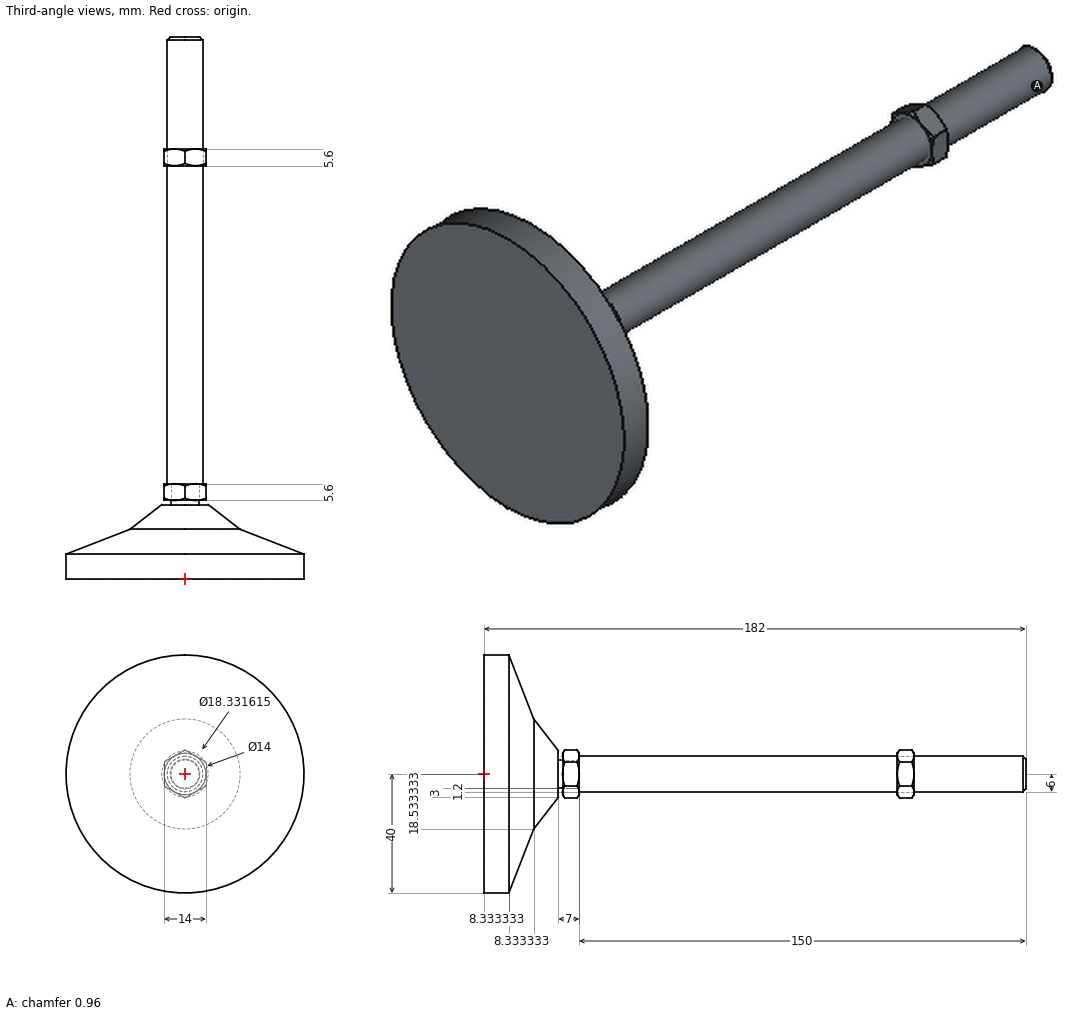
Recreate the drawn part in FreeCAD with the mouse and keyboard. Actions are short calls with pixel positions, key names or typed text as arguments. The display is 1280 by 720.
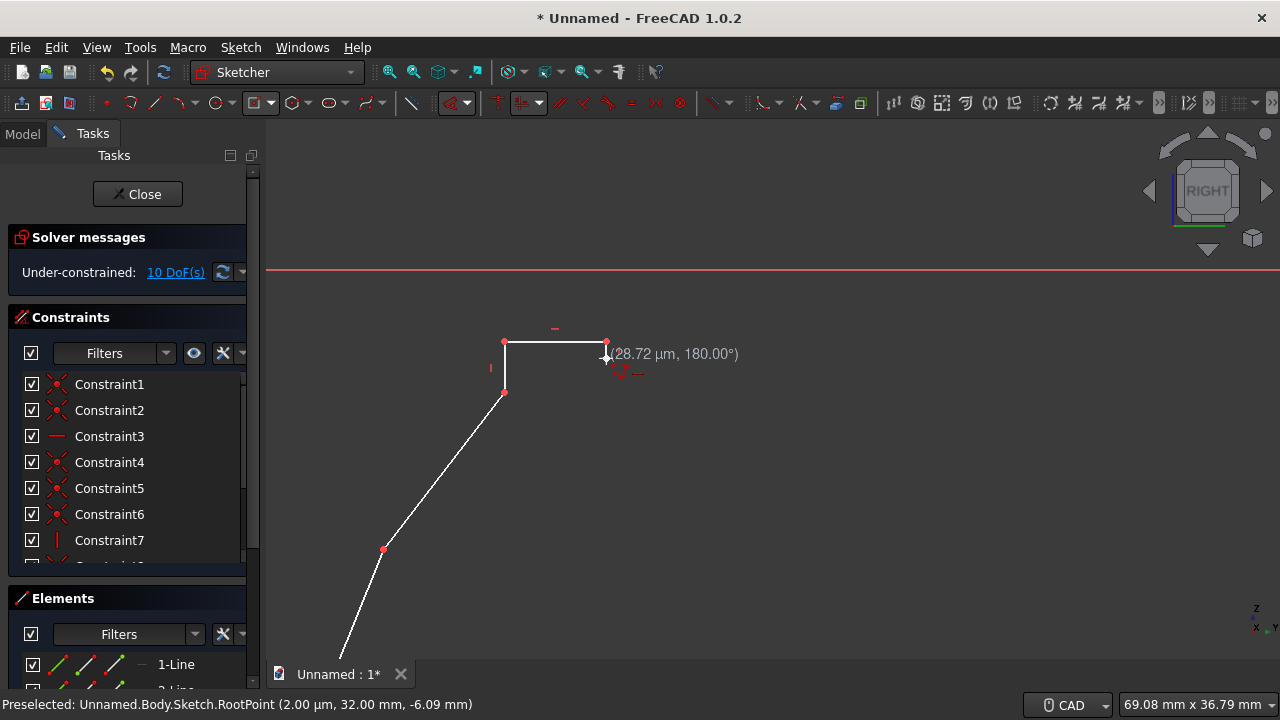
scroll(510, 345, down, 8)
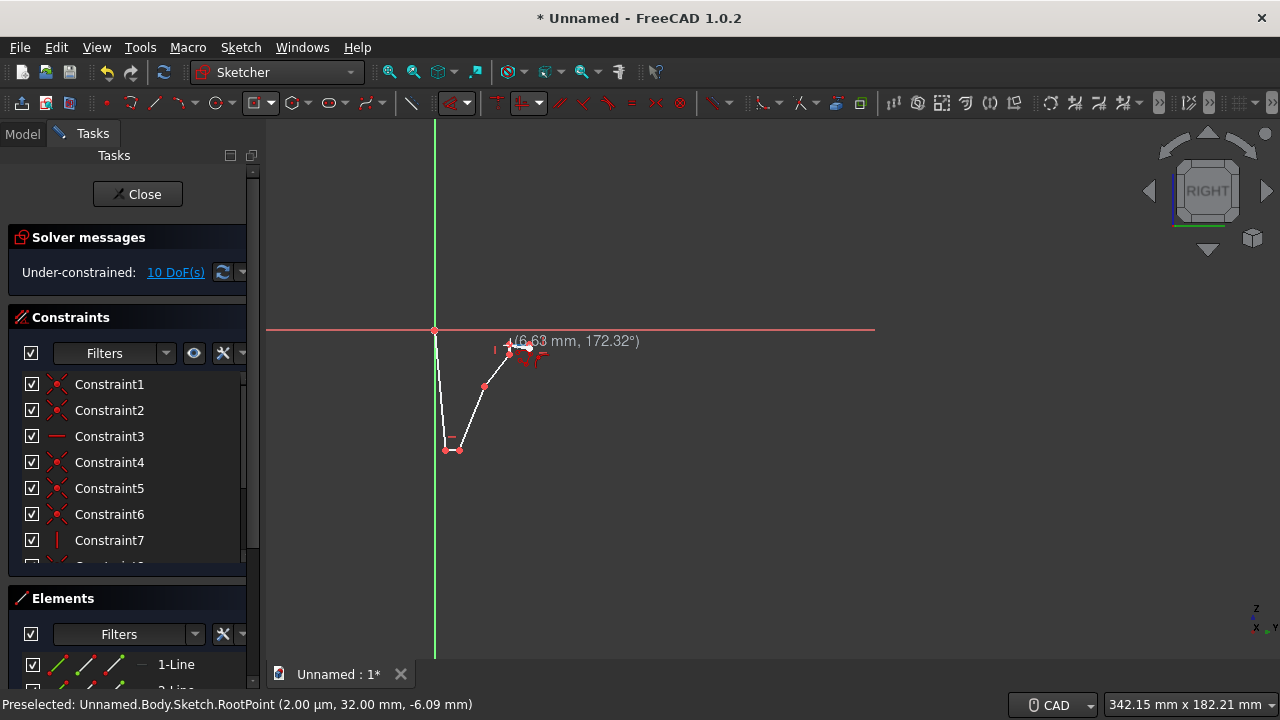
click(974, 348)
click(974, 339)
click(435, 330)
key(Escape)
key(Escape)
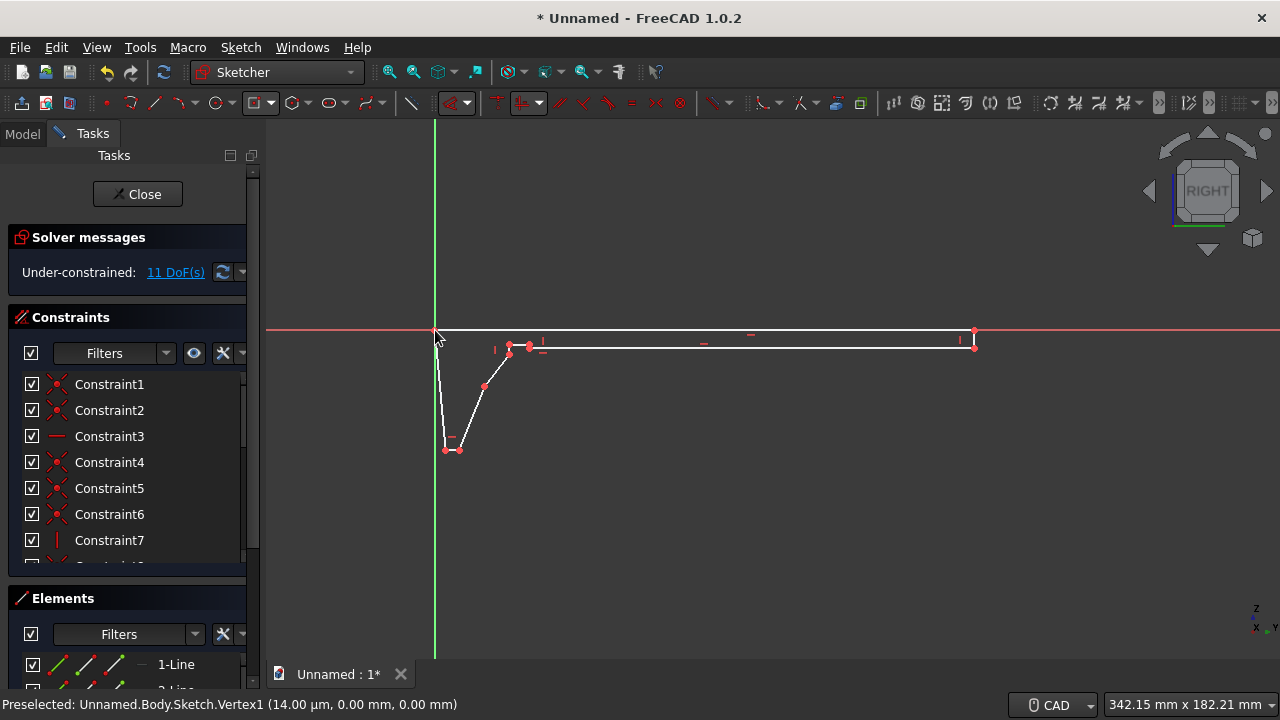
click(438, 366)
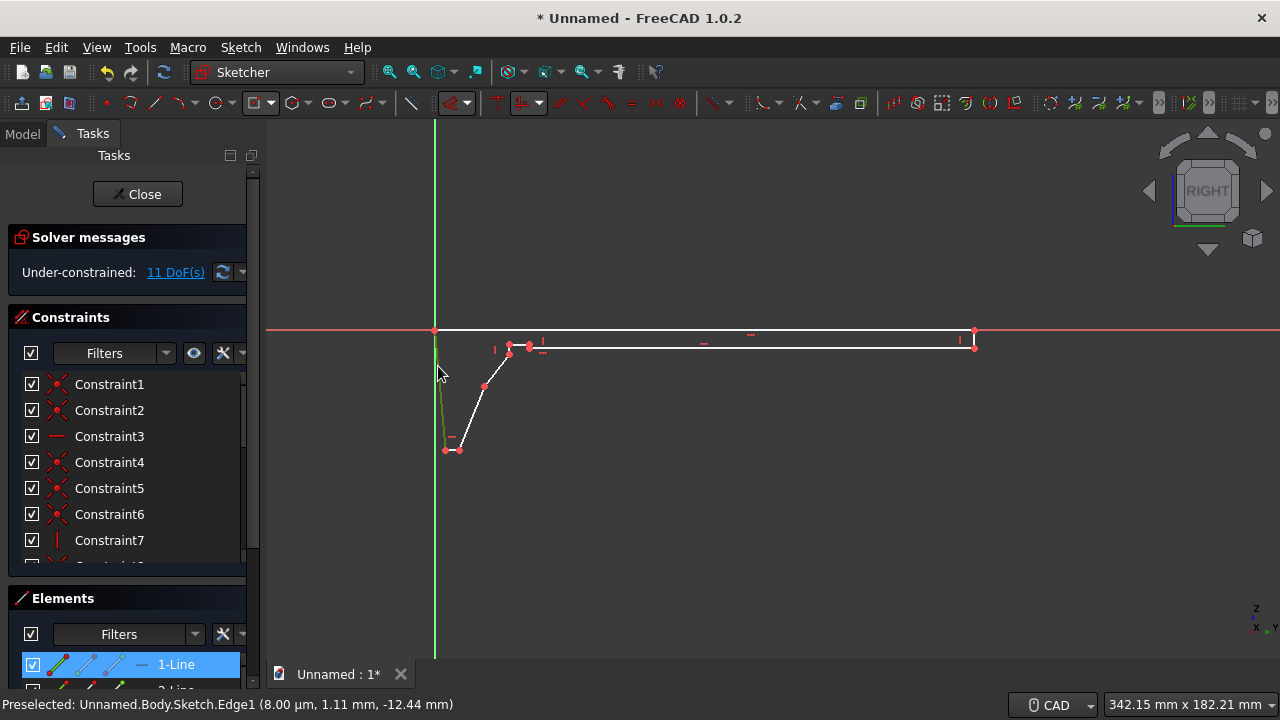
key(v)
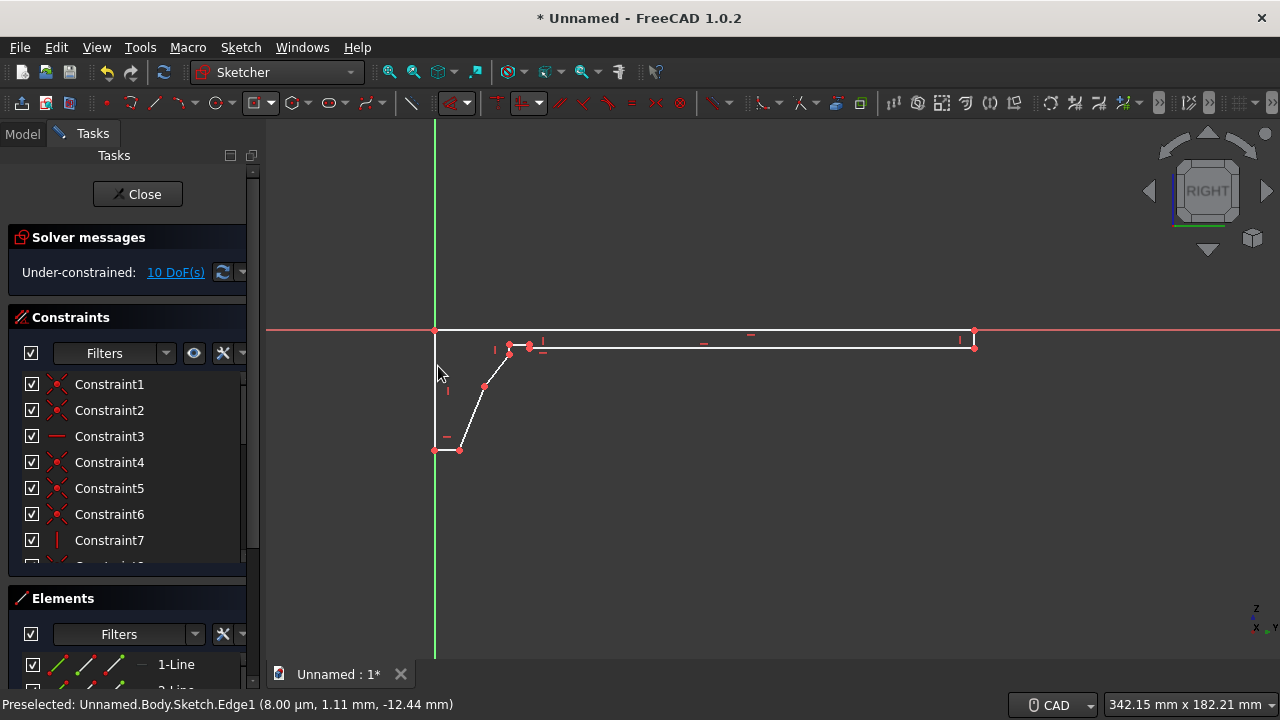
click(450, 104)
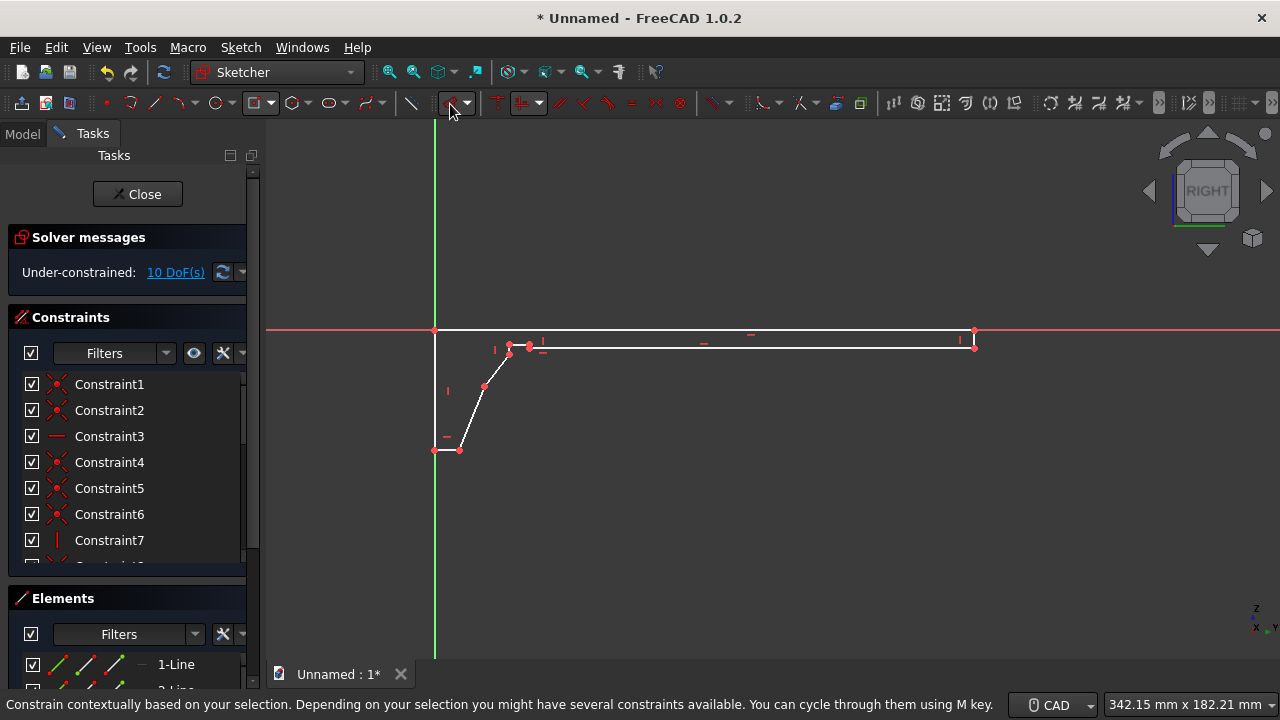
scroll(509, 350, up, 8)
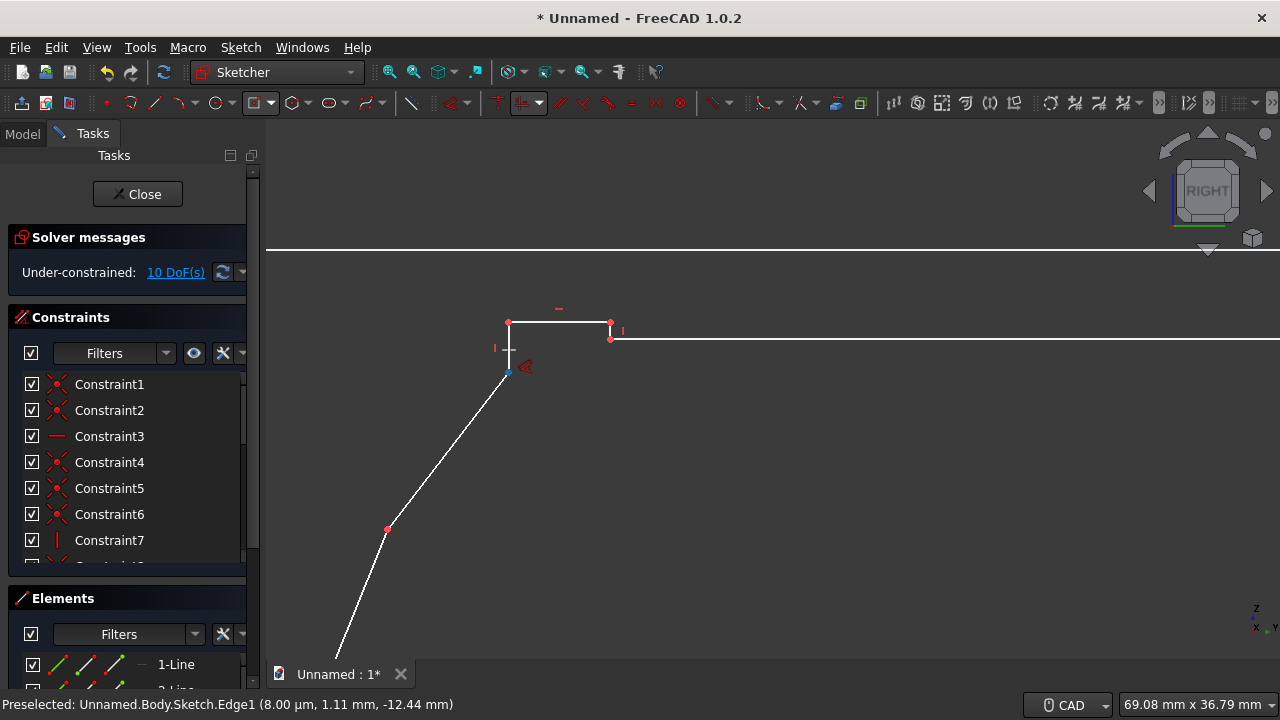
click(509, 347)
click(475, 347)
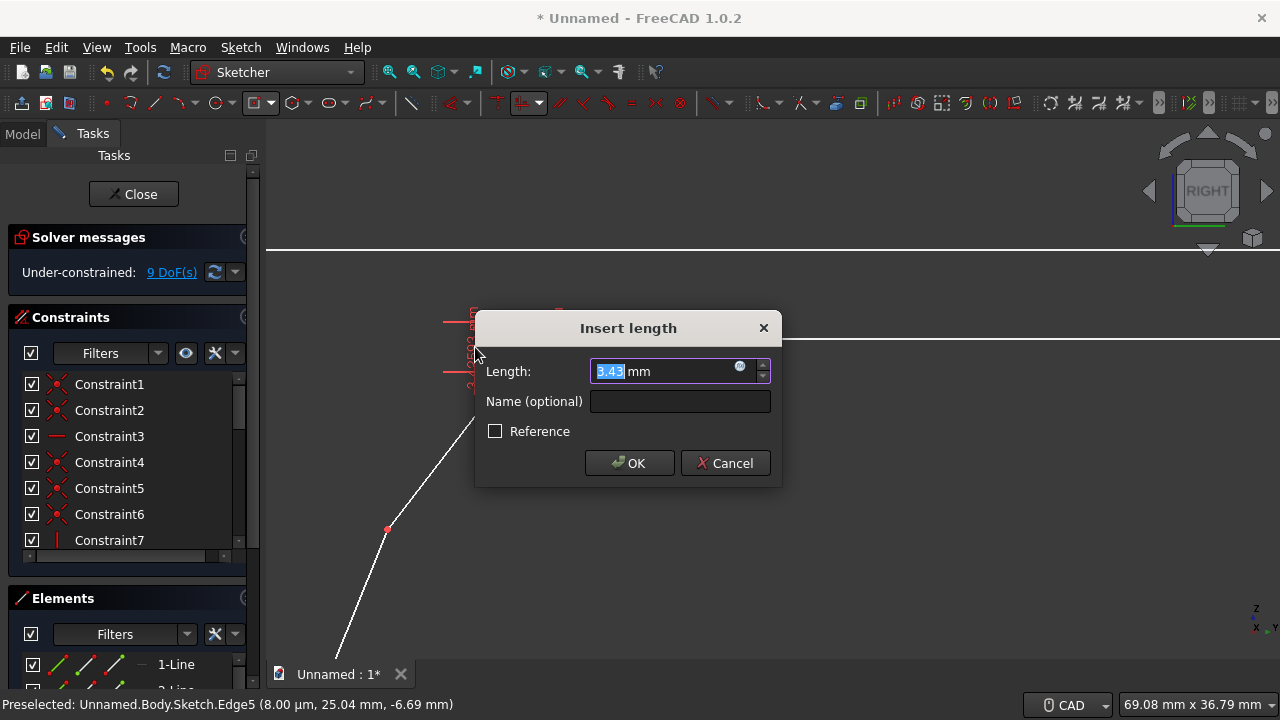
text(3)
key(Return)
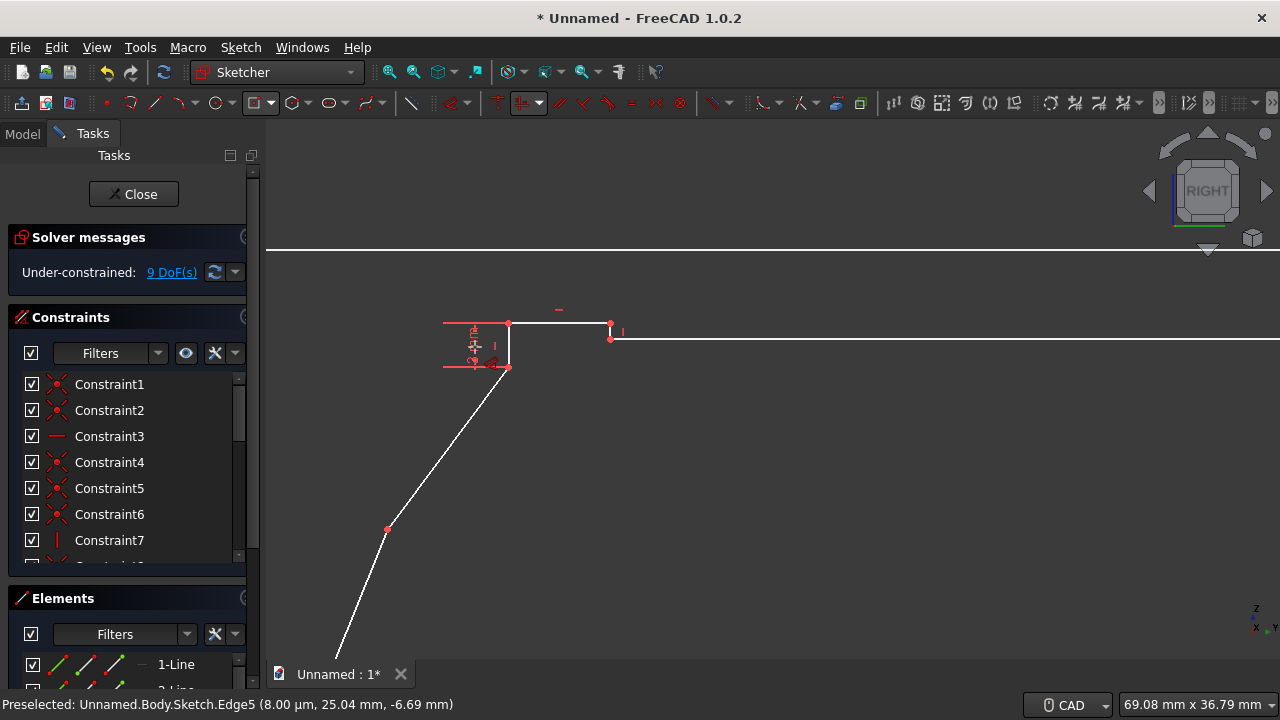
click(539, 323)
click(560, 289)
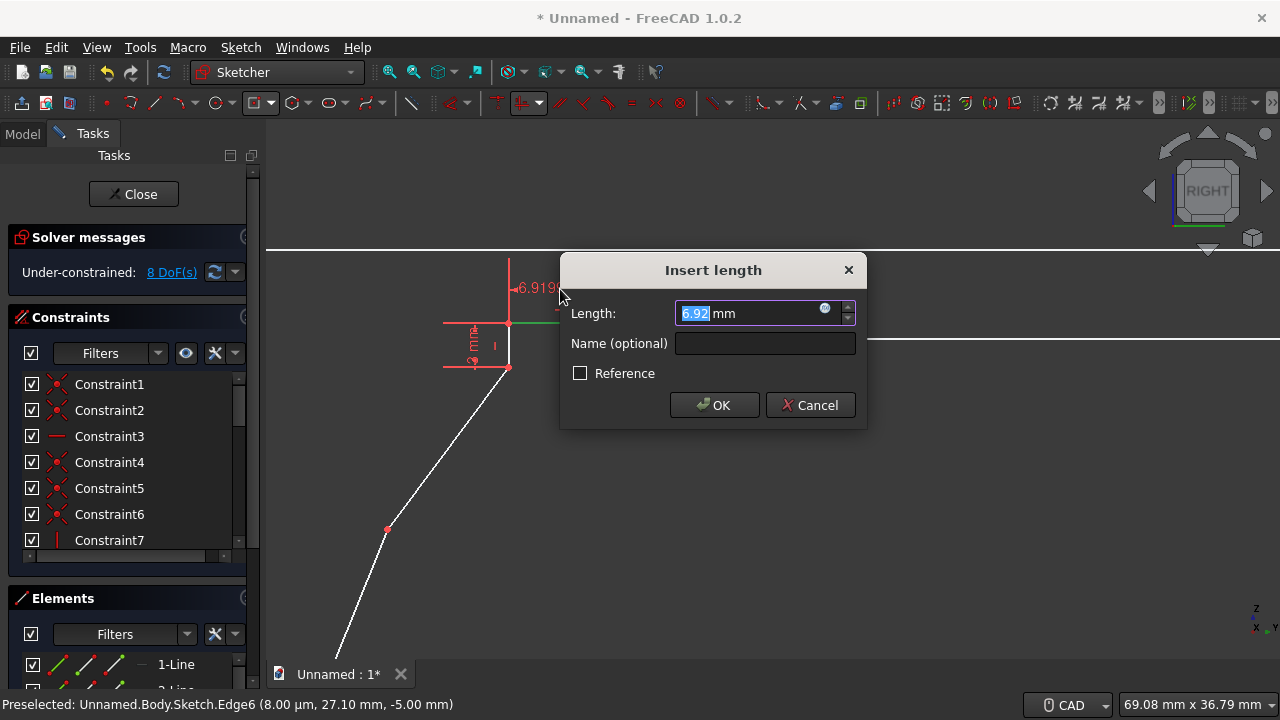
text(7)
key(Return)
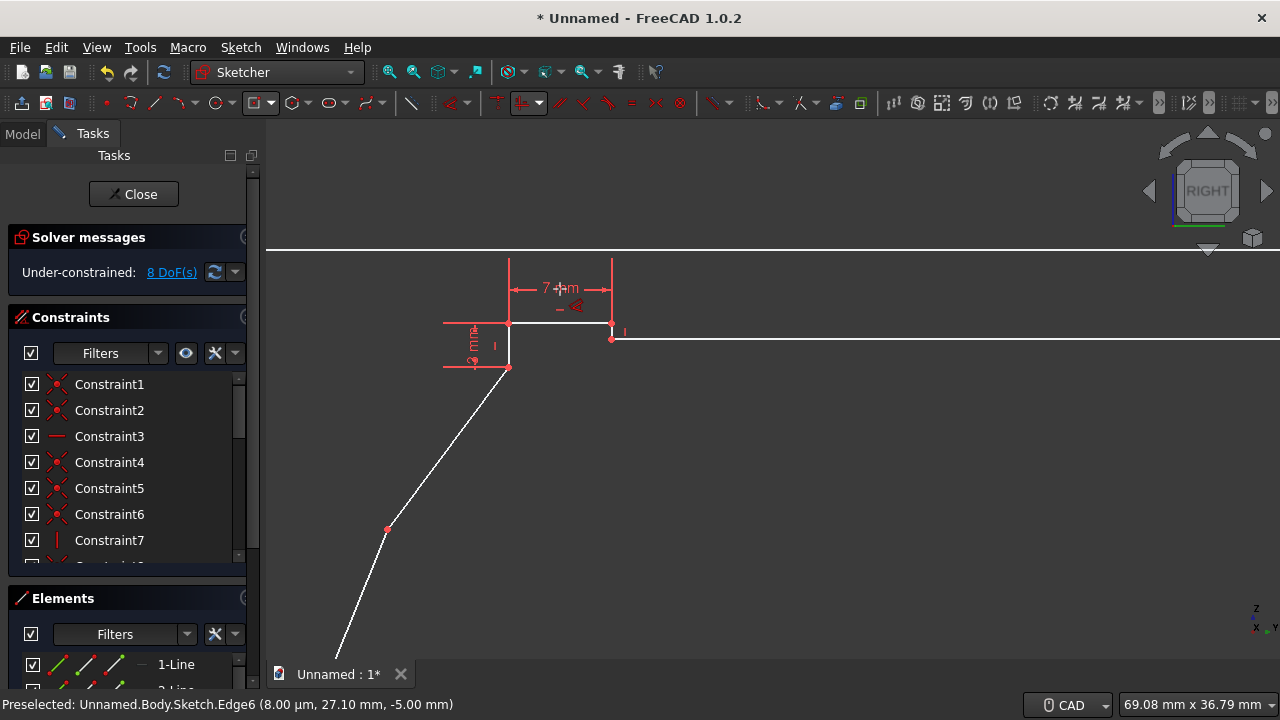
scroll(509, 350, down, 8)